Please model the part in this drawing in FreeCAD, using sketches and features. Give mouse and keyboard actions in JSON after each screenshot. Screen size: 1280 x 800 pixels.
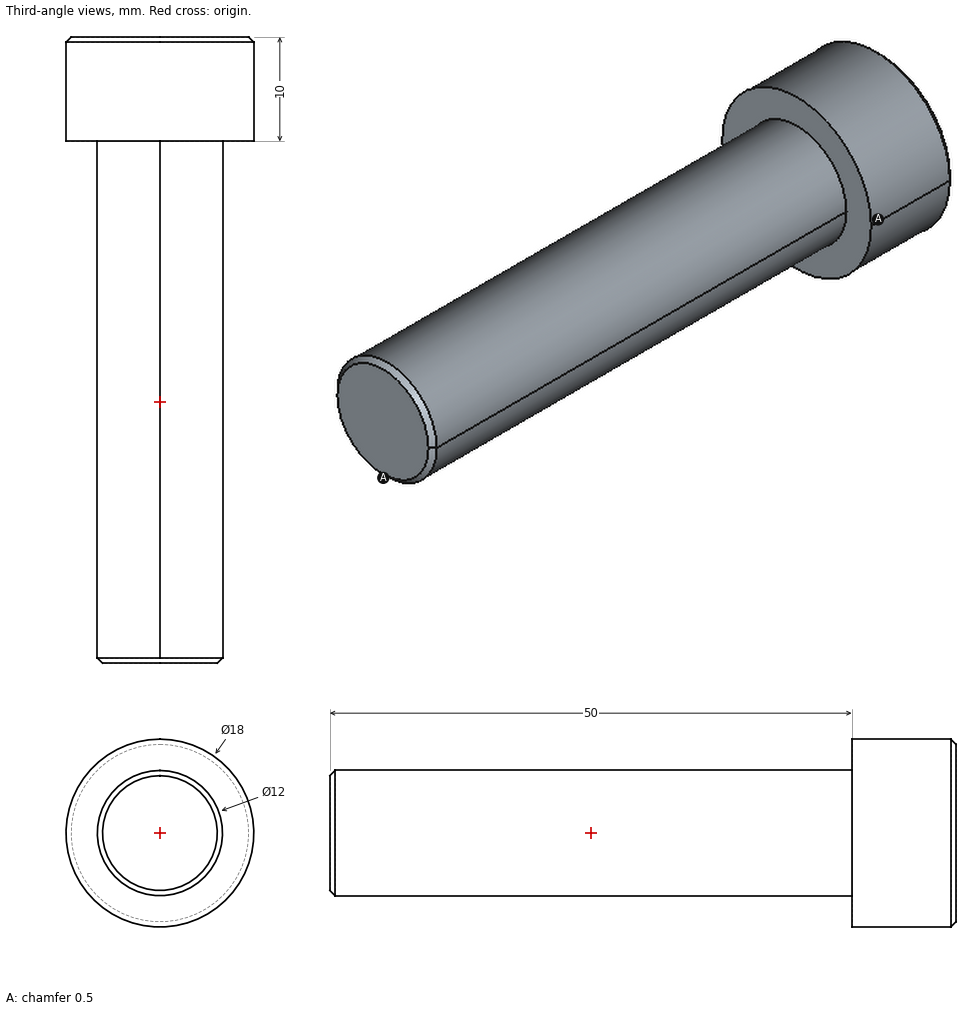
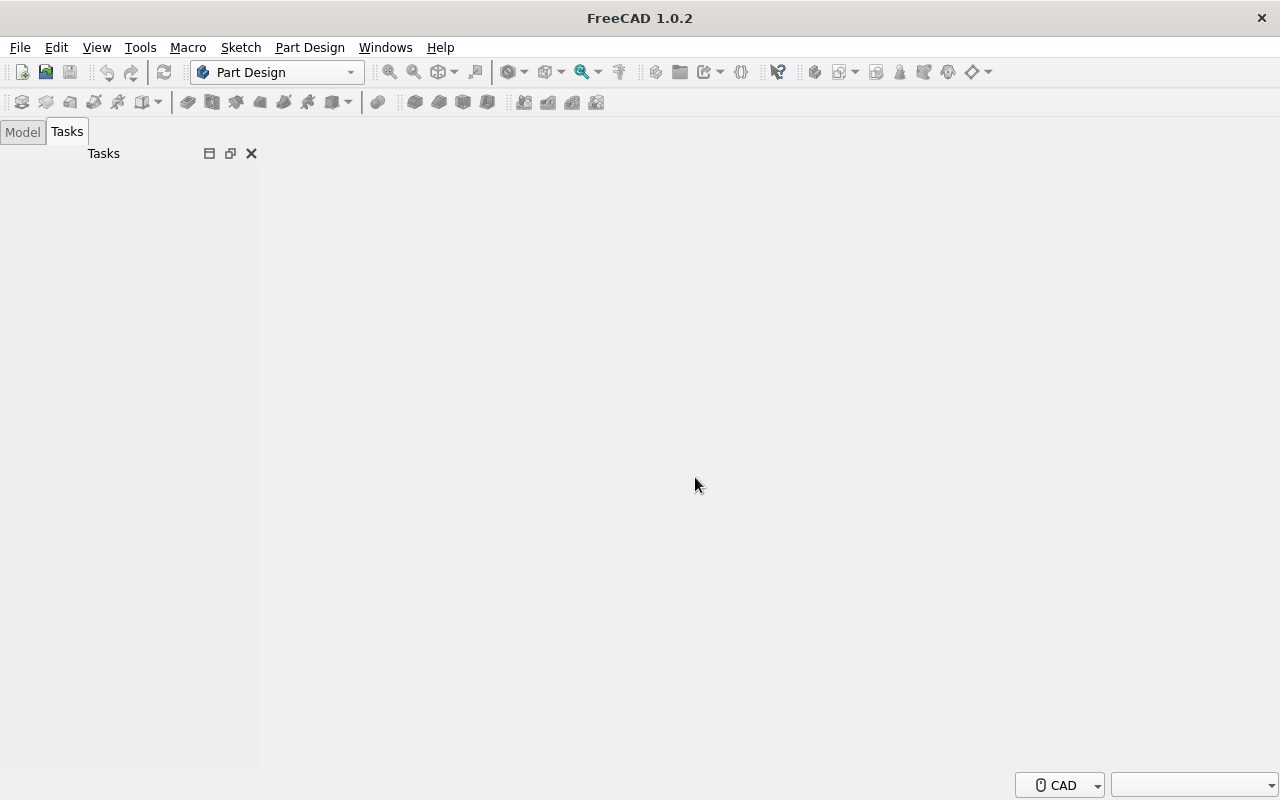
{"action": "left_click", "coordinate": [22, 72]}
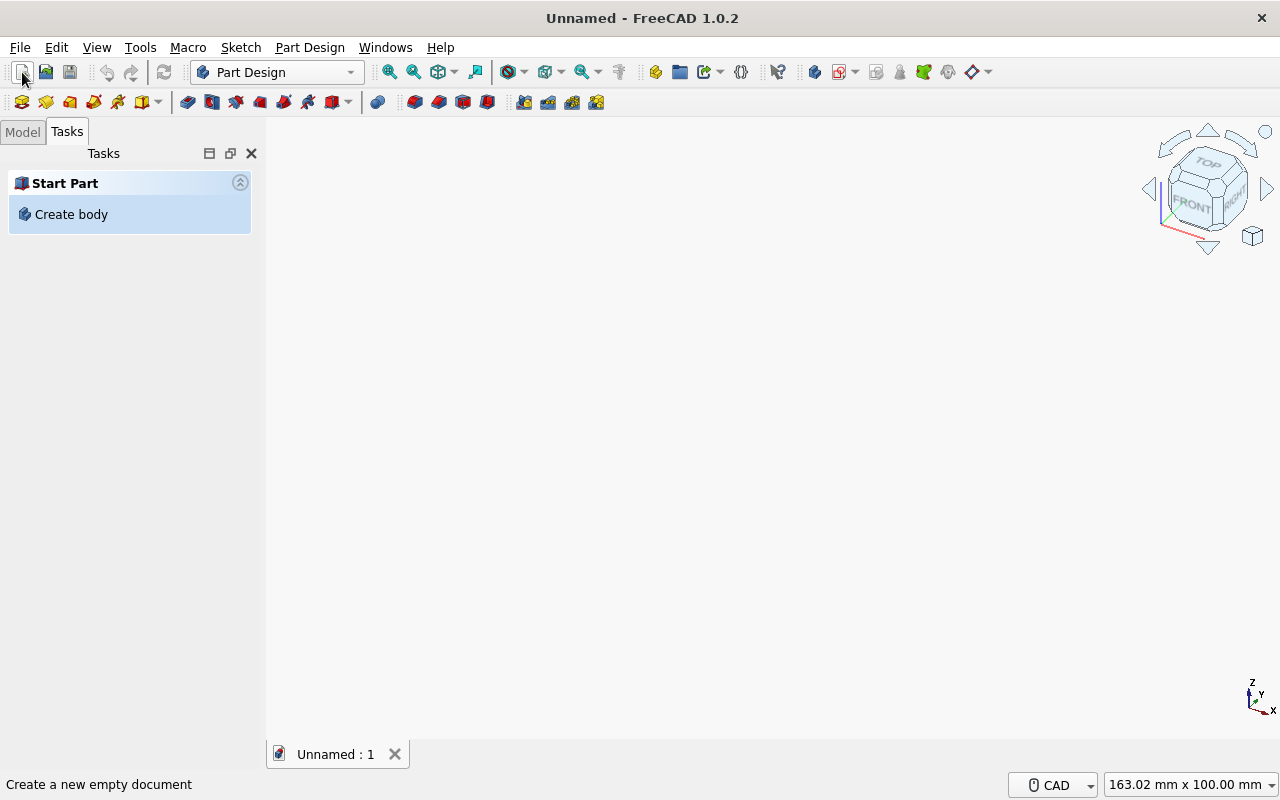
{"action": "left_click", "coordinate": [840, 72]}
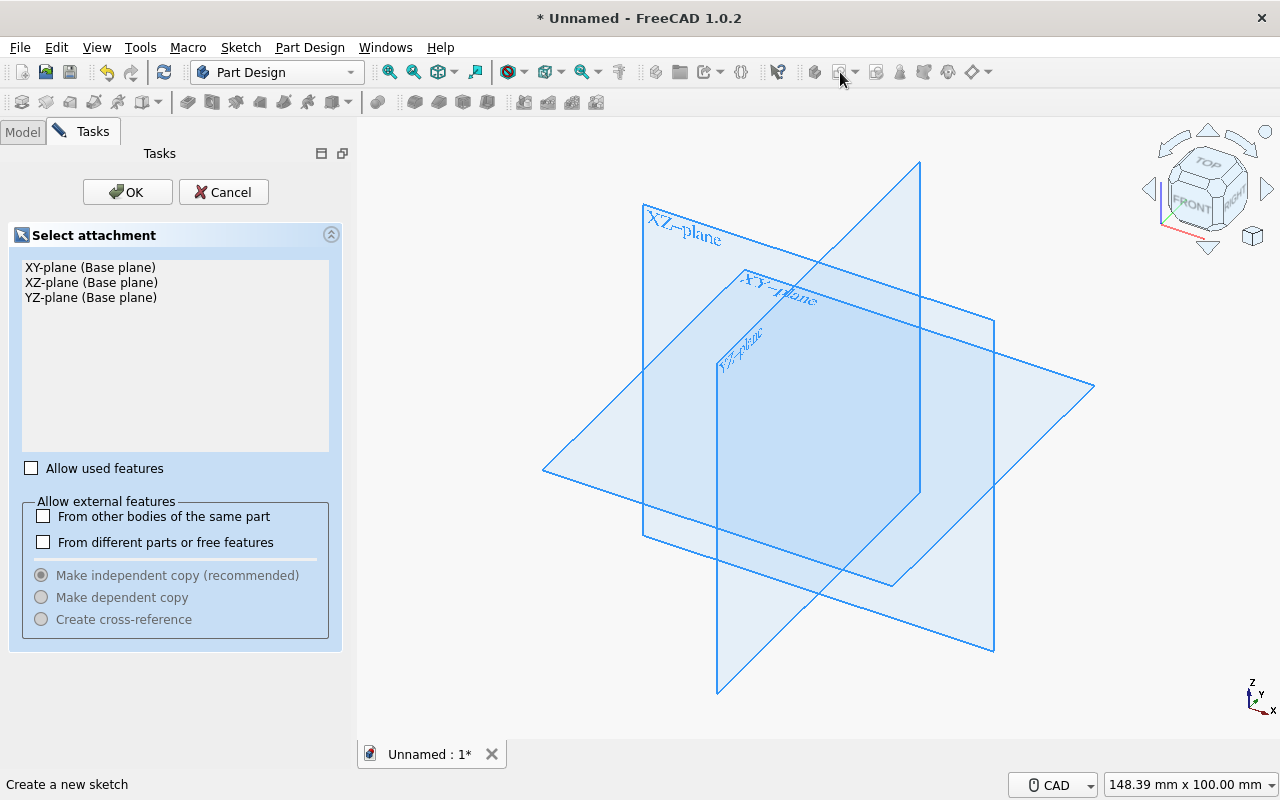
{"action": "left_click", "coordinate": [82, 282]}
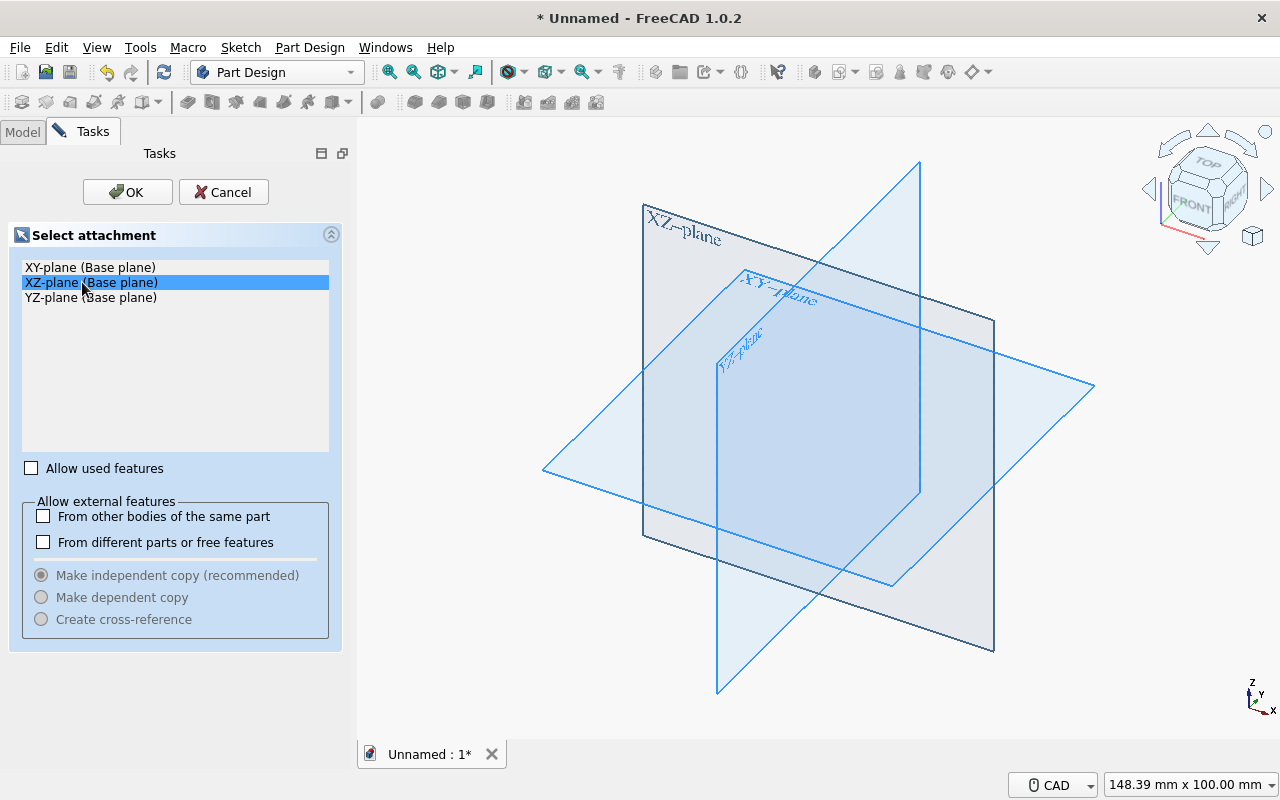
{"action": "left_click", "coordinate": [128, 192]}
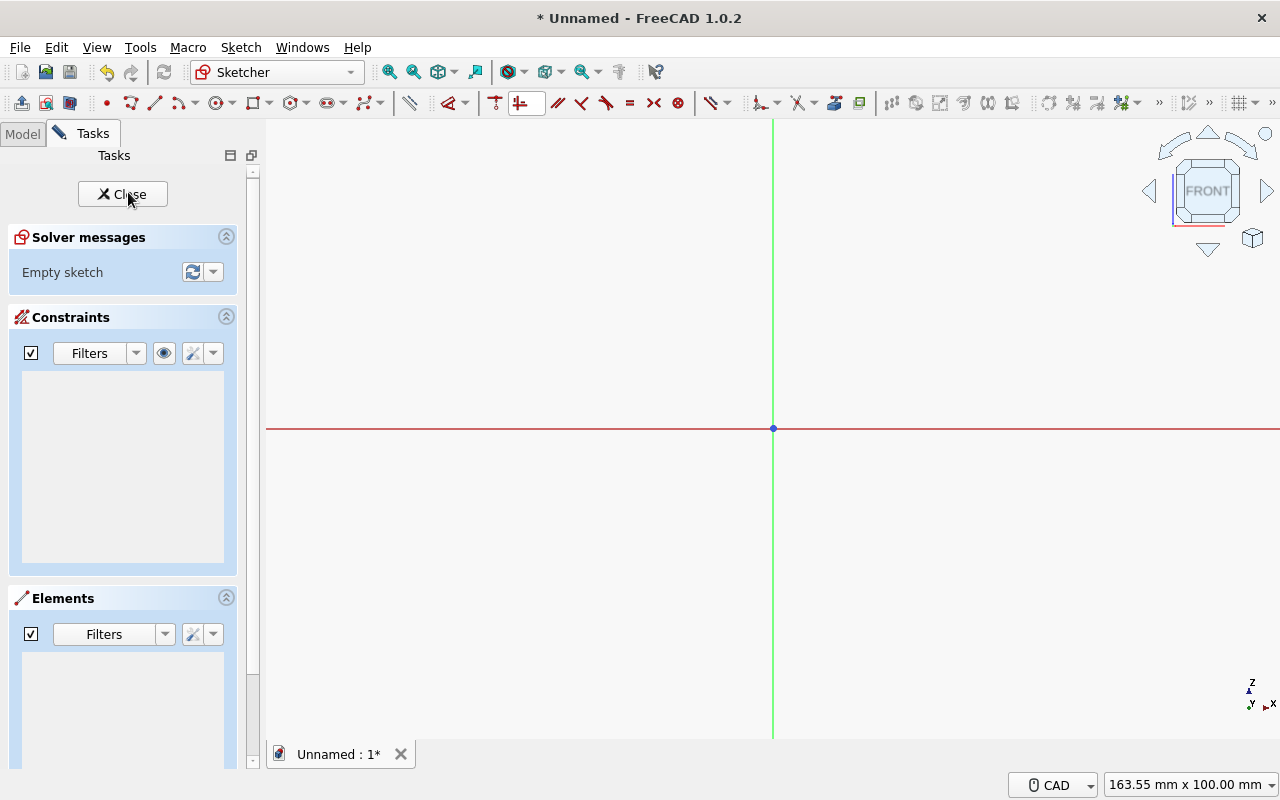
{"action": "scroll", "coordinate": [790, 429], "scroll_direction": "up", "scroll_amount": 8}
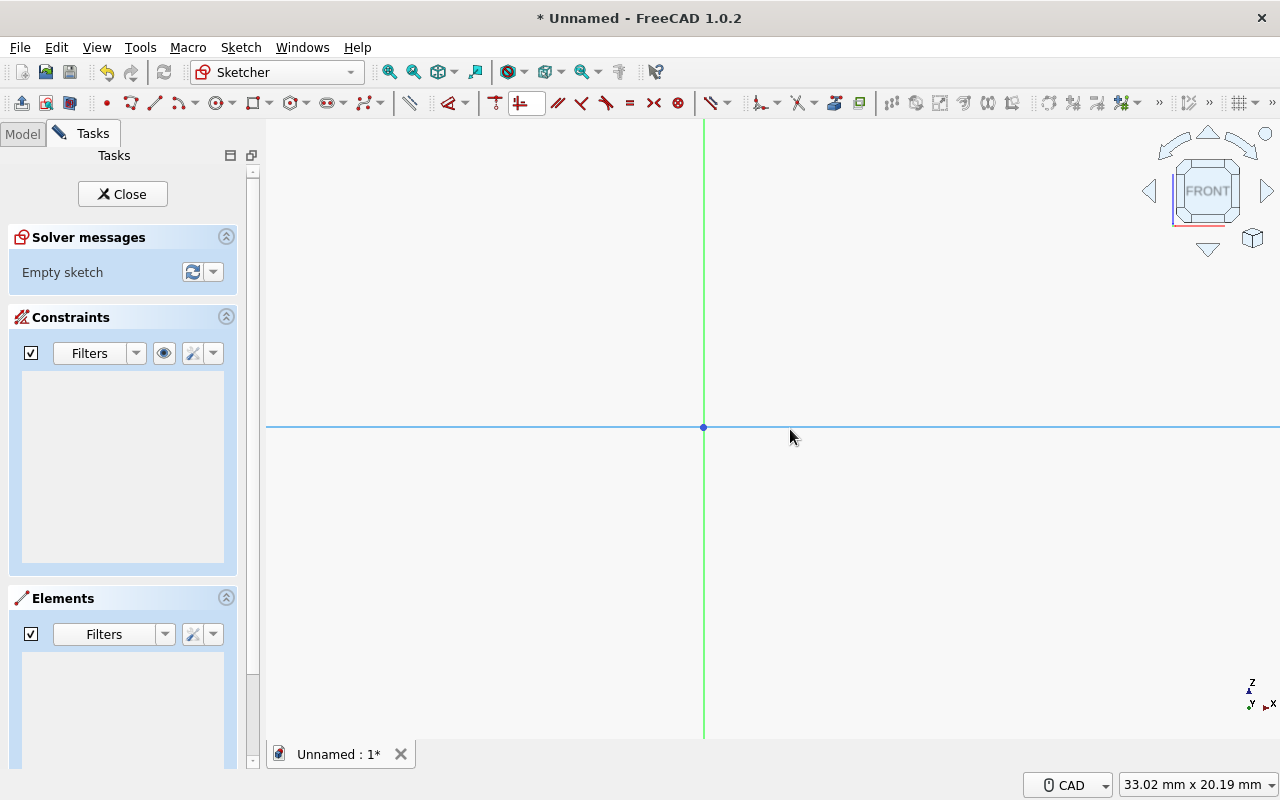
{"action": "left_click", "coordinate": [216, 104]}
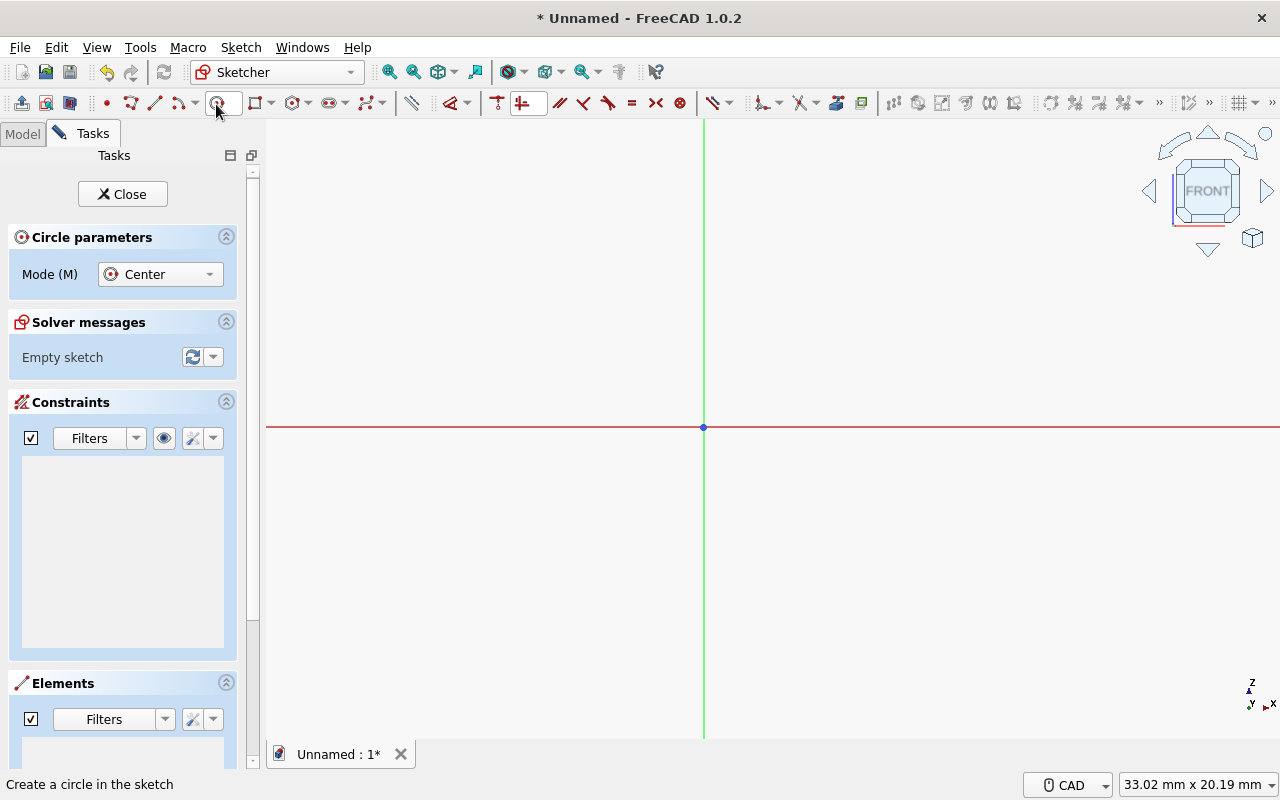
{"action": "left_click", "coordinate": [704, 427]}
{"action": "left_click", "coordinate": [834, 297]}
{"action": "key", "text": "Escape"}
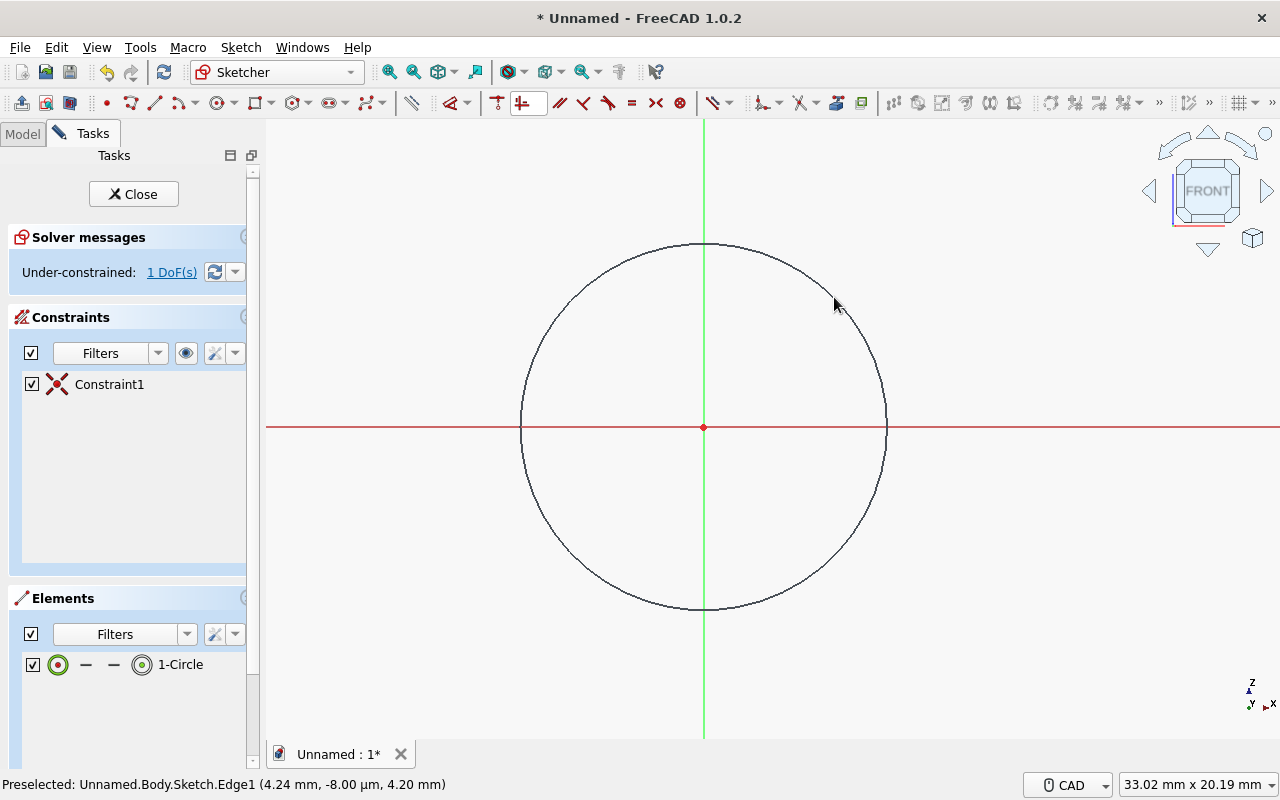
{"action": "left_click", "coordinate": [833, 297]}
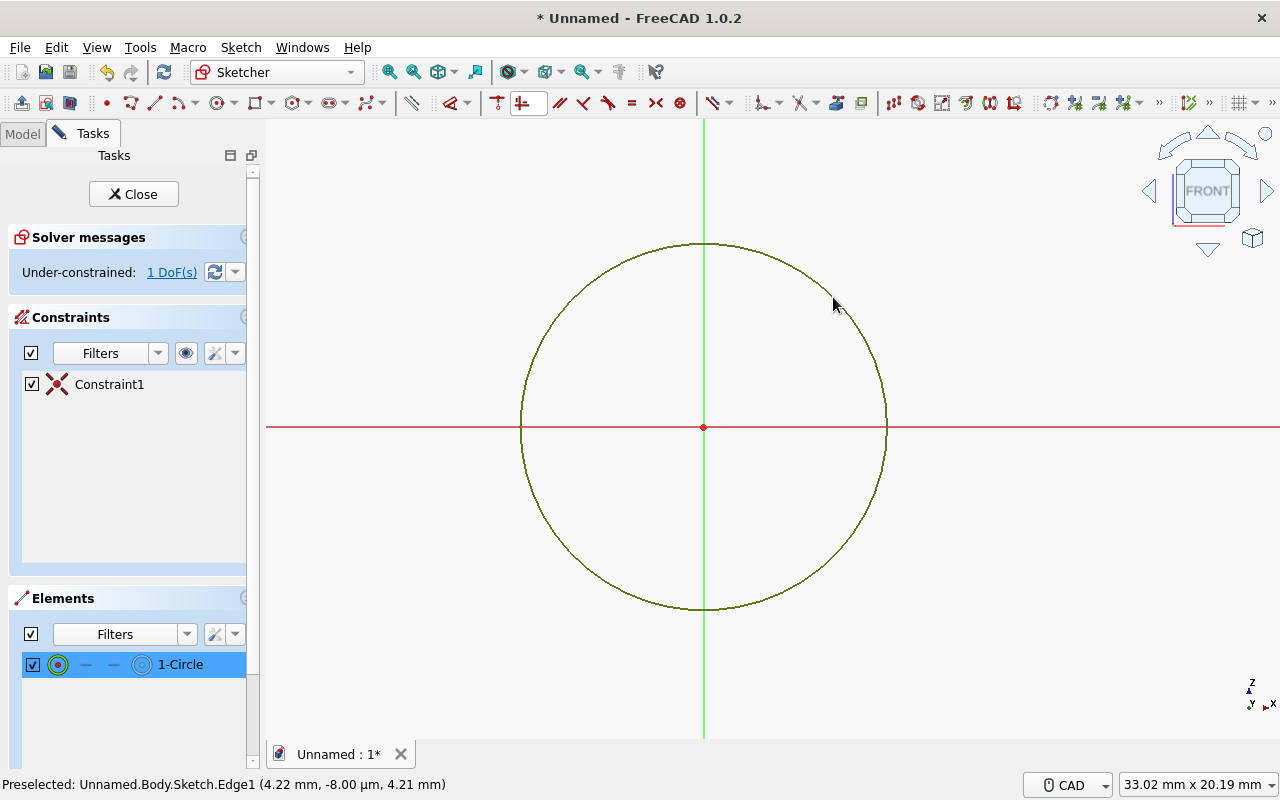
{"action": "left_click", "coordinate": [470, 104]}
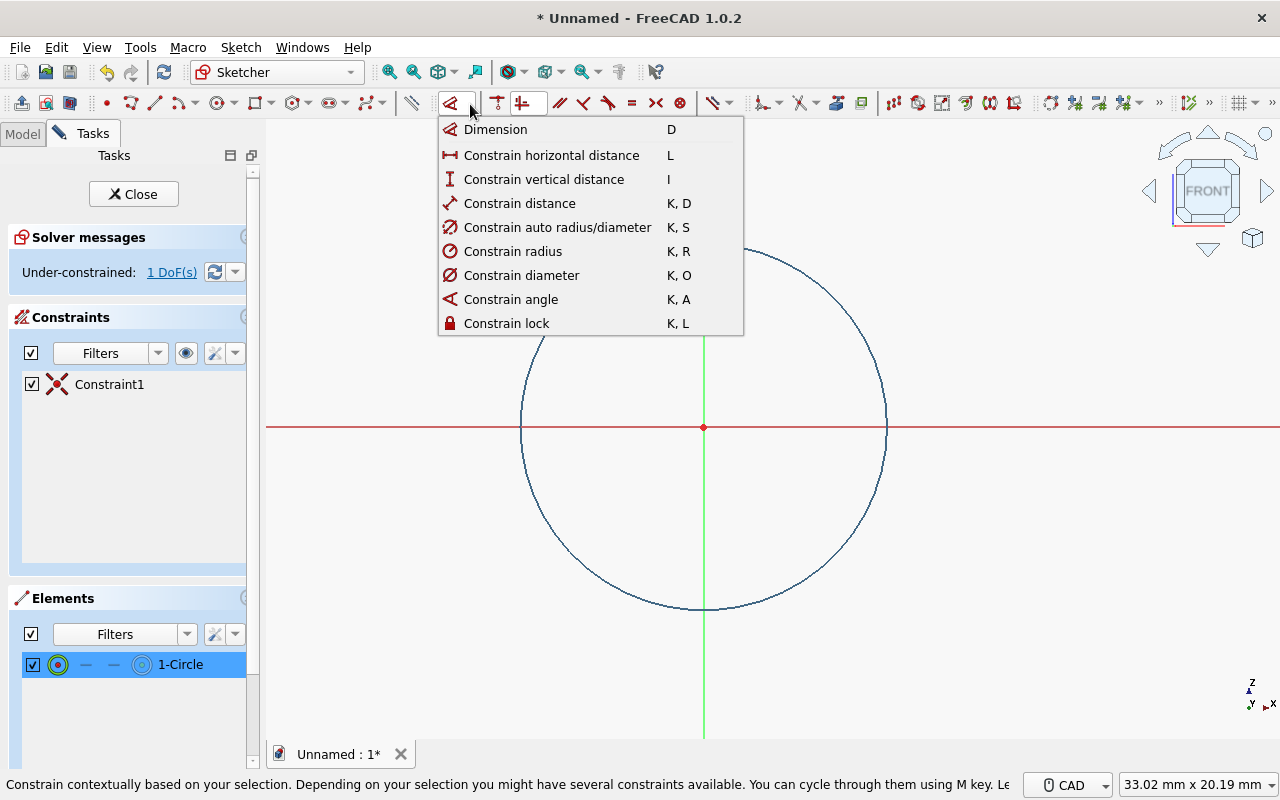
{"action": "left_click", "coordinate": [591, 275]}